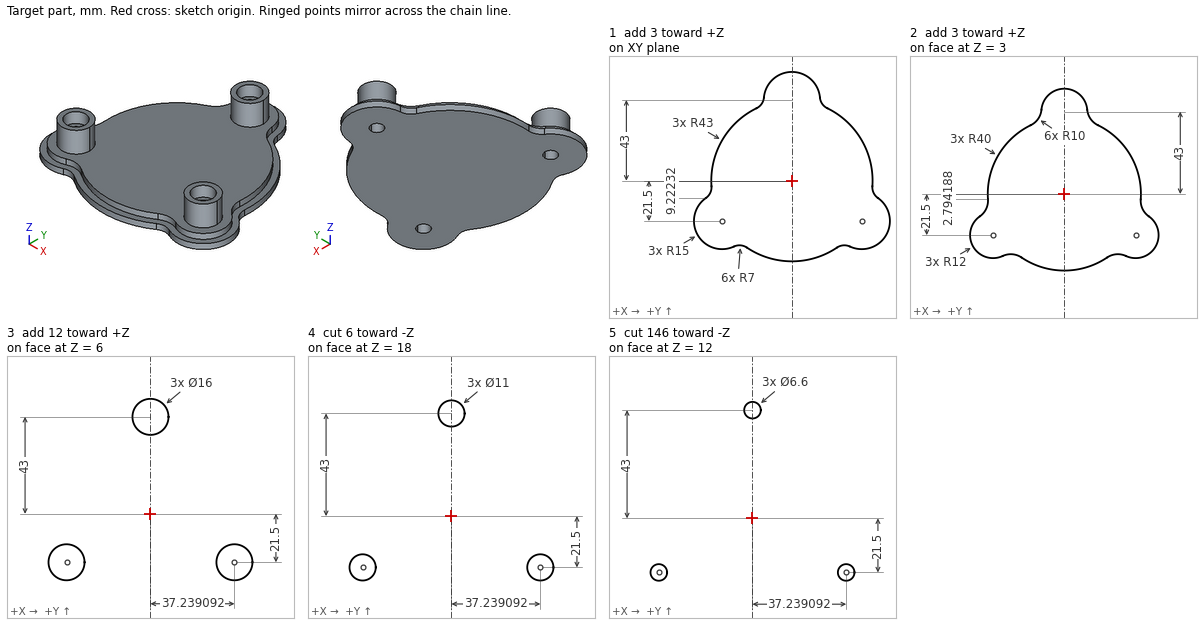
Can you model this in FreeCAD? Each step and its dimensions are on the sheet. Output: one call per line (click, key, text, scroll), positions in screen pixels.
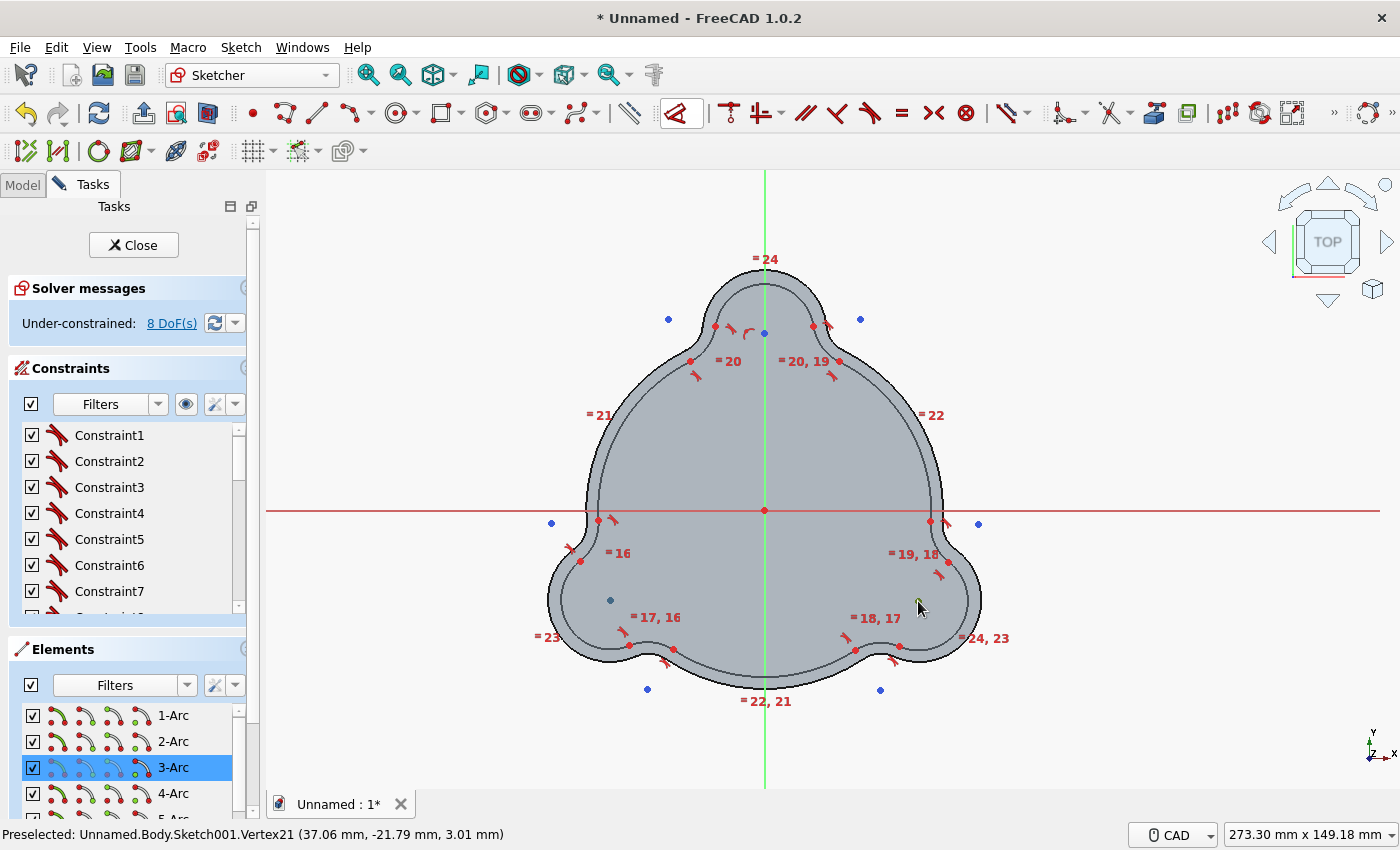
click(765, 721)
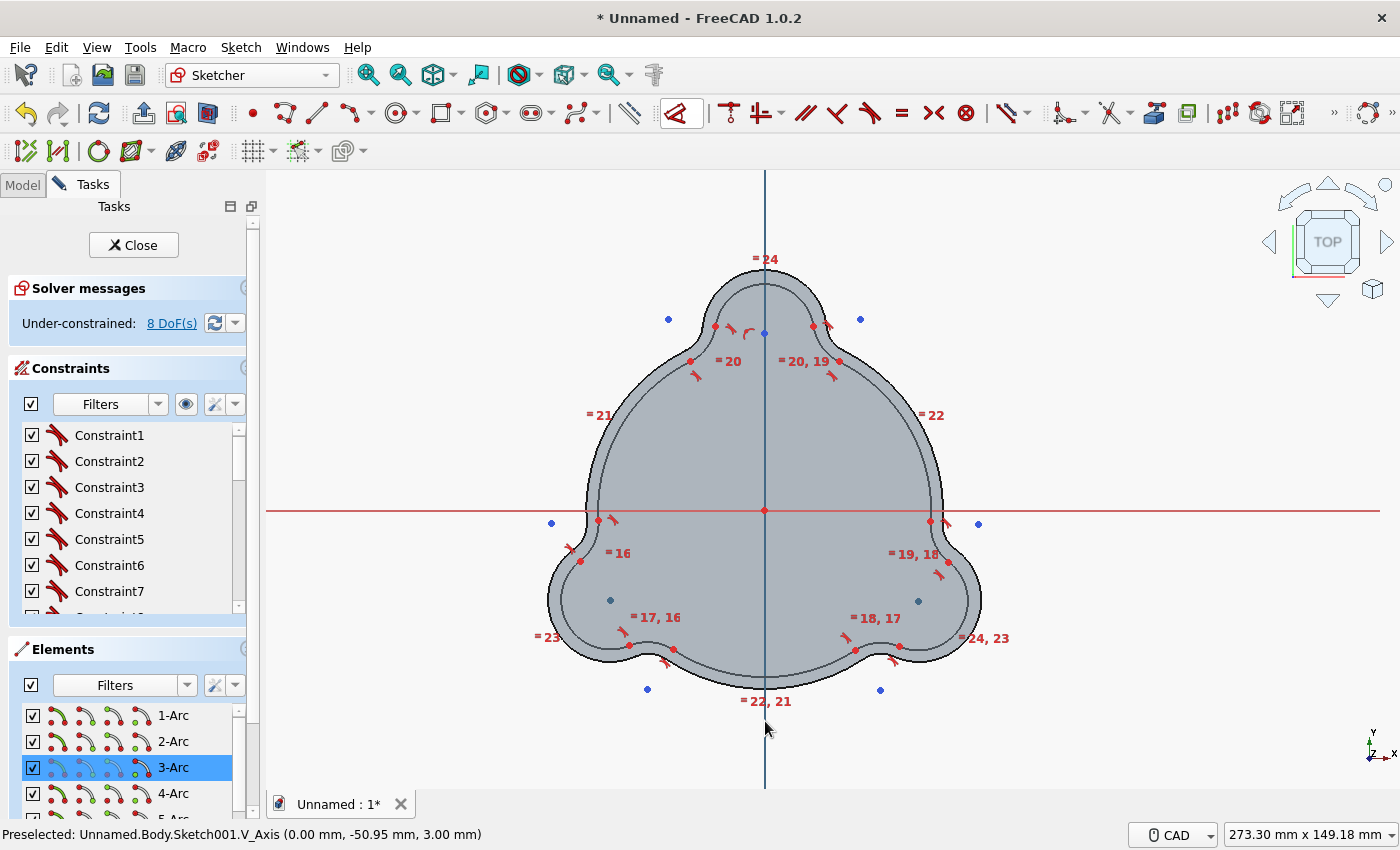
click(934, 114)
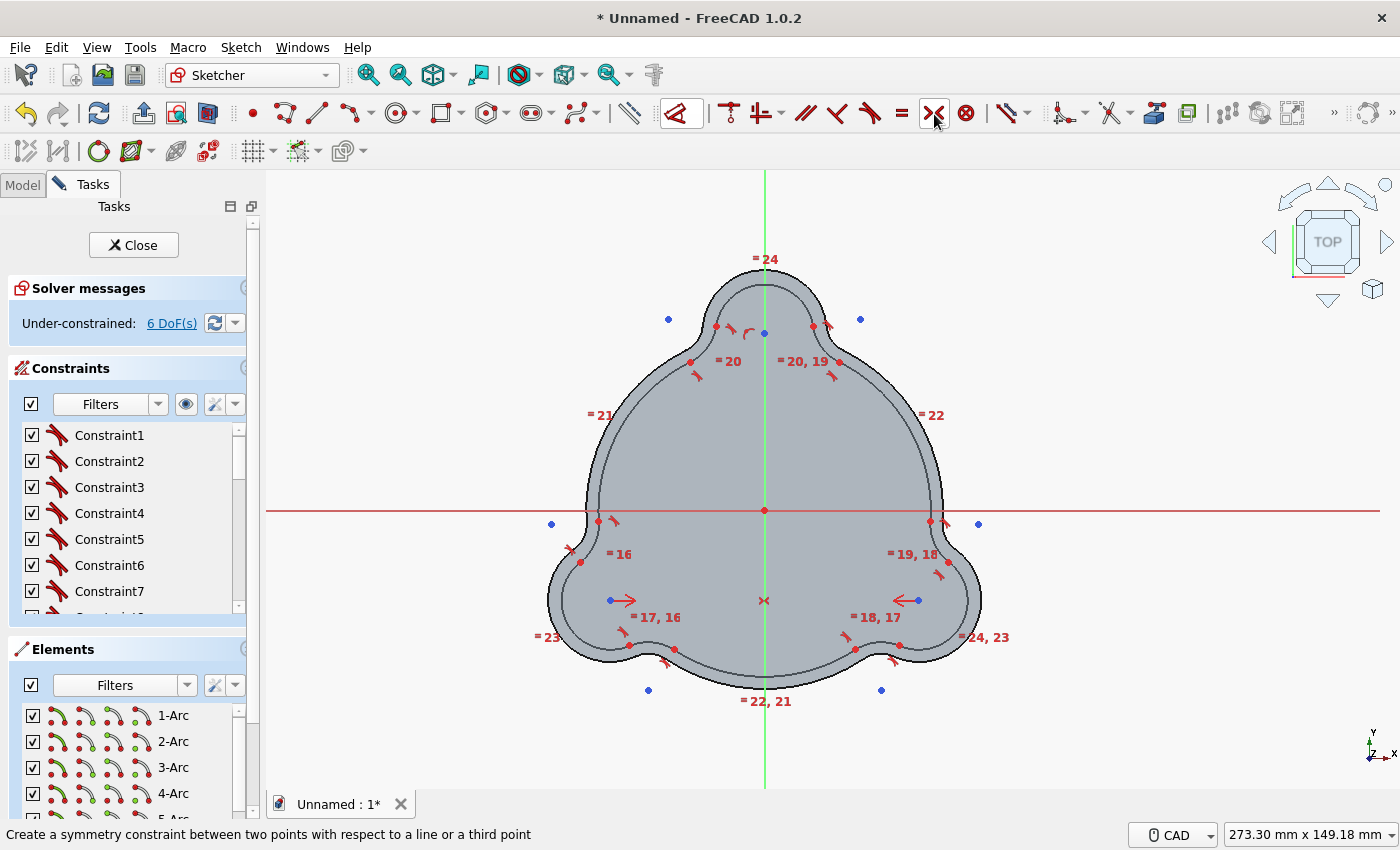
click(644, 397)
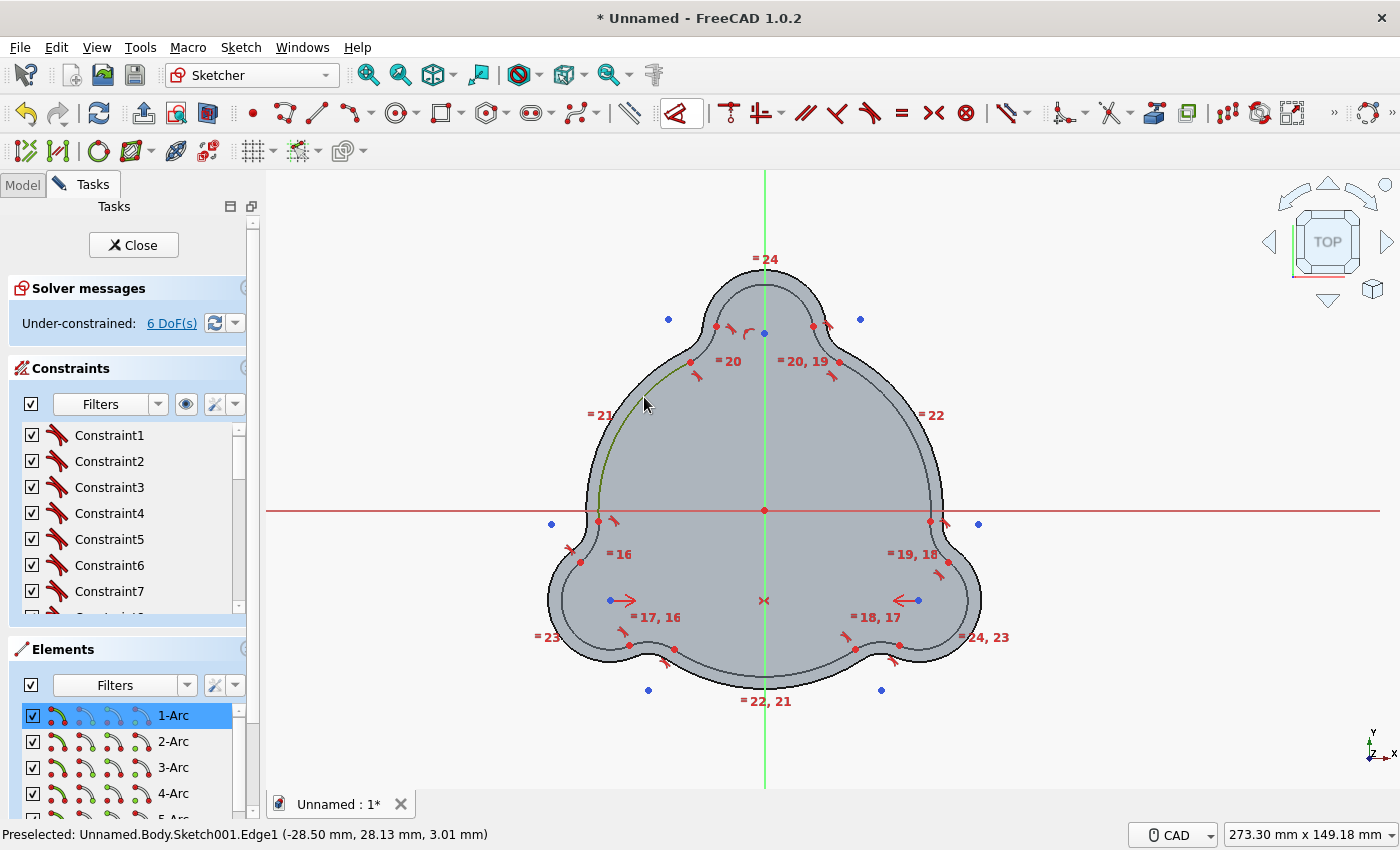
click(698, 114)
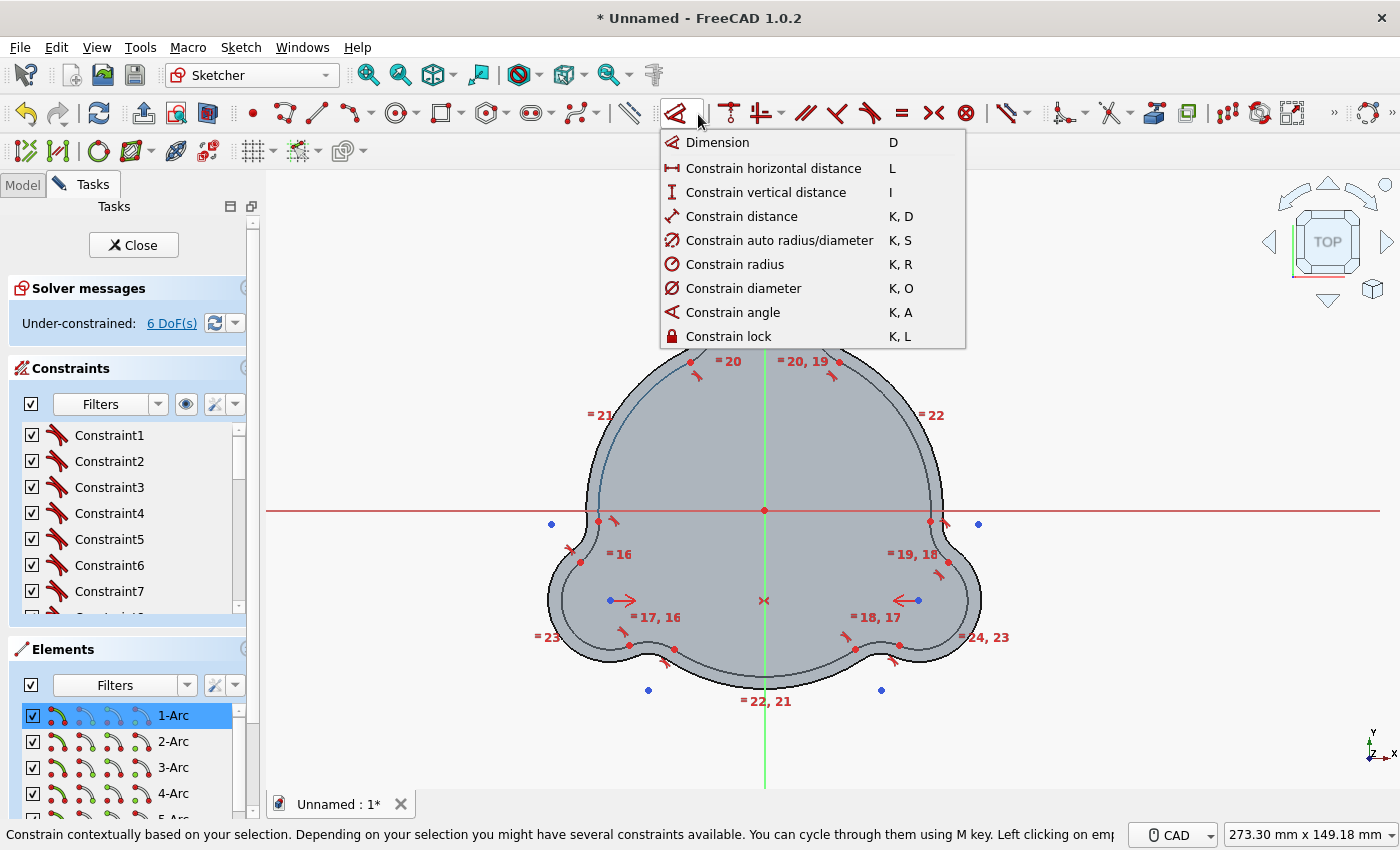
click(813, 264)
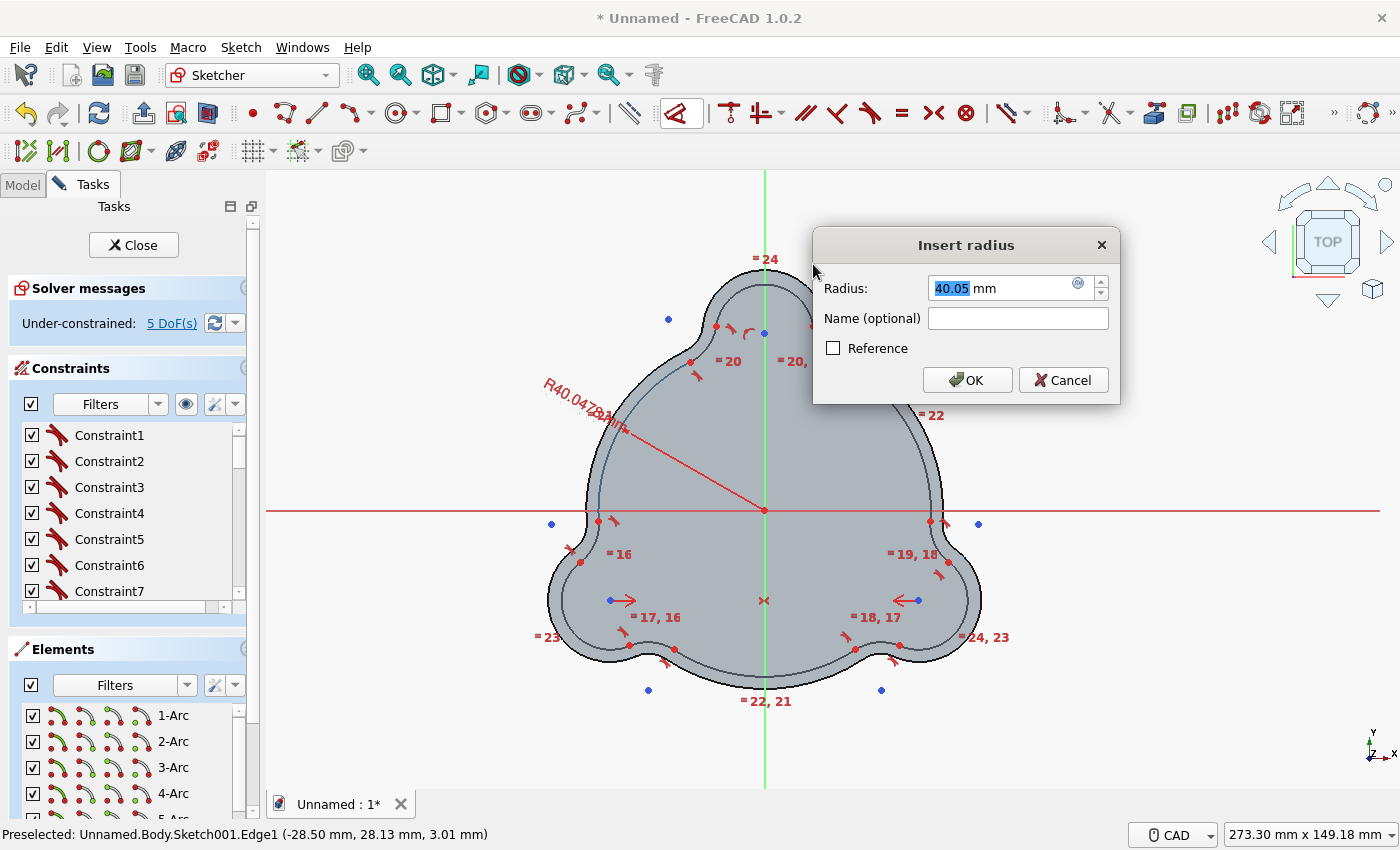
text(40)
key(Return)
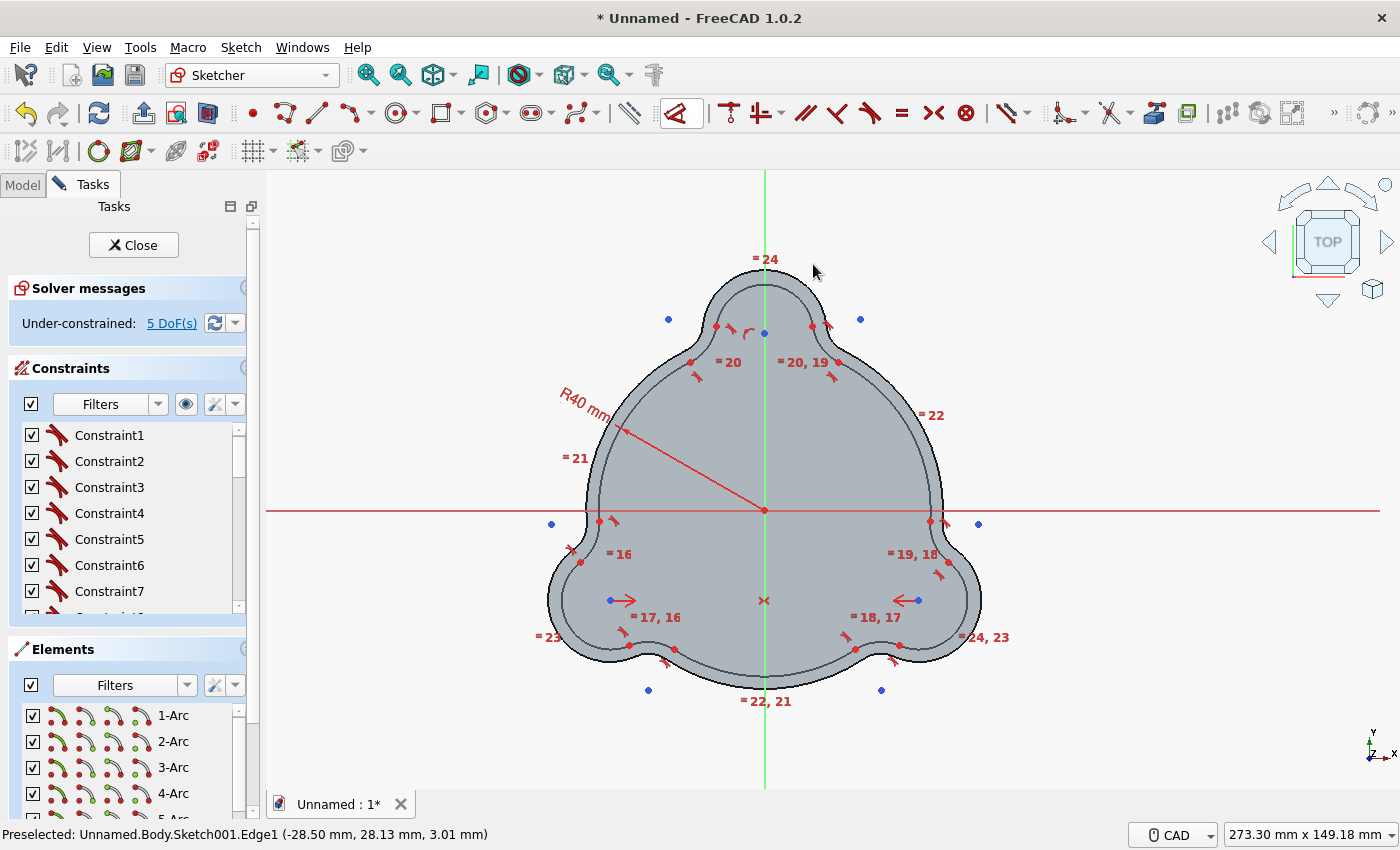
click(590, 552)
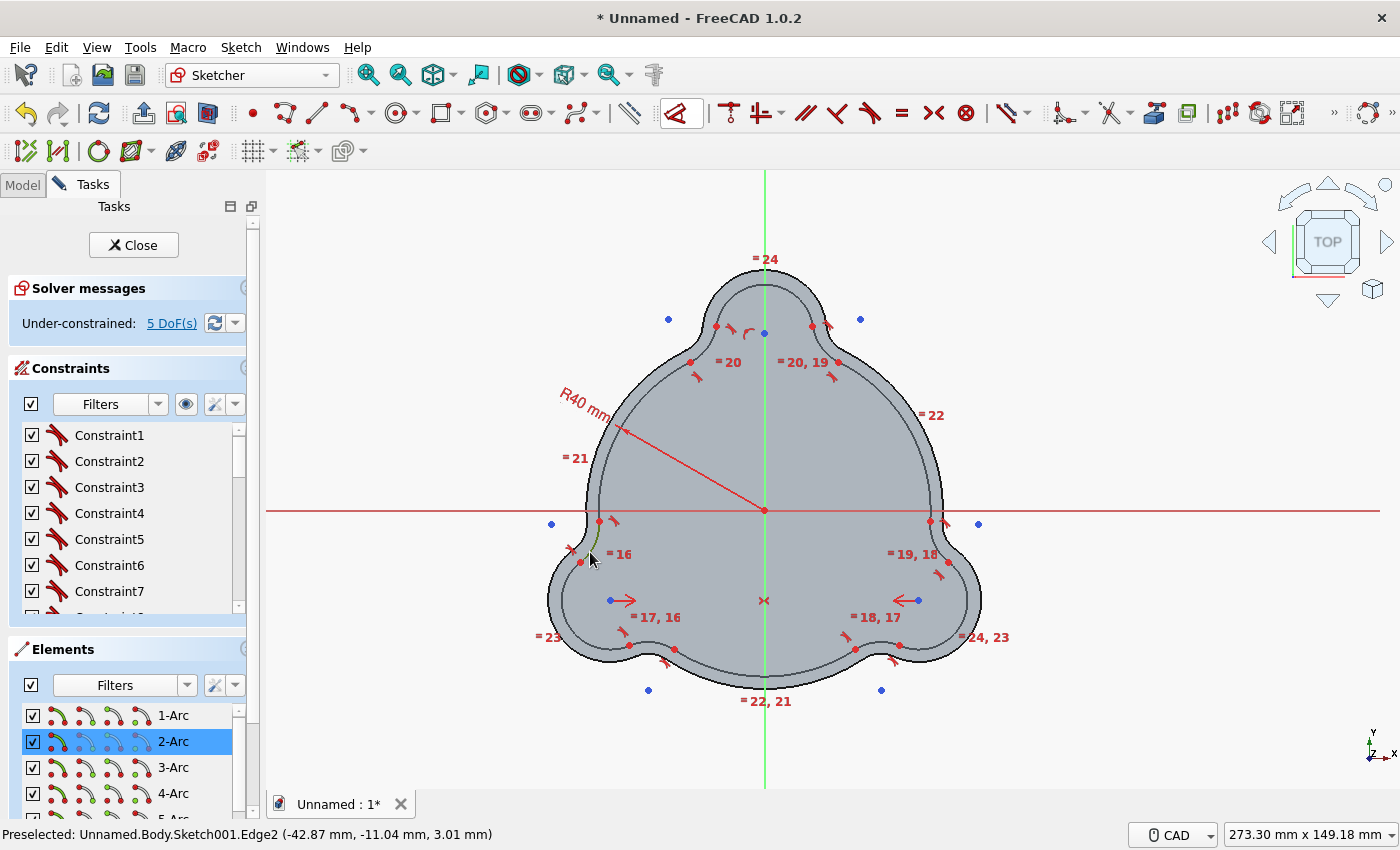
key(k)
key(r)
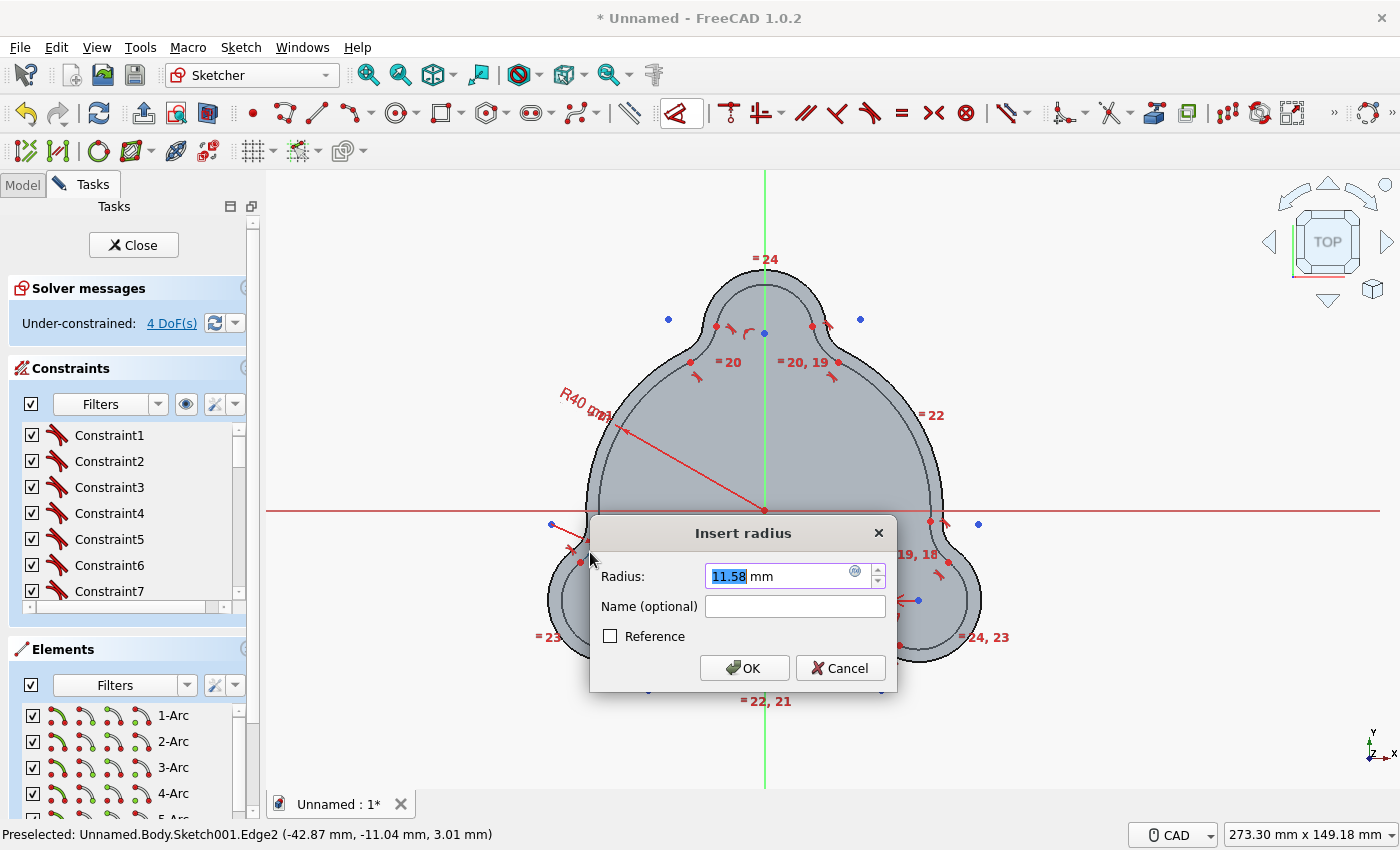
text(10)
key(Return)